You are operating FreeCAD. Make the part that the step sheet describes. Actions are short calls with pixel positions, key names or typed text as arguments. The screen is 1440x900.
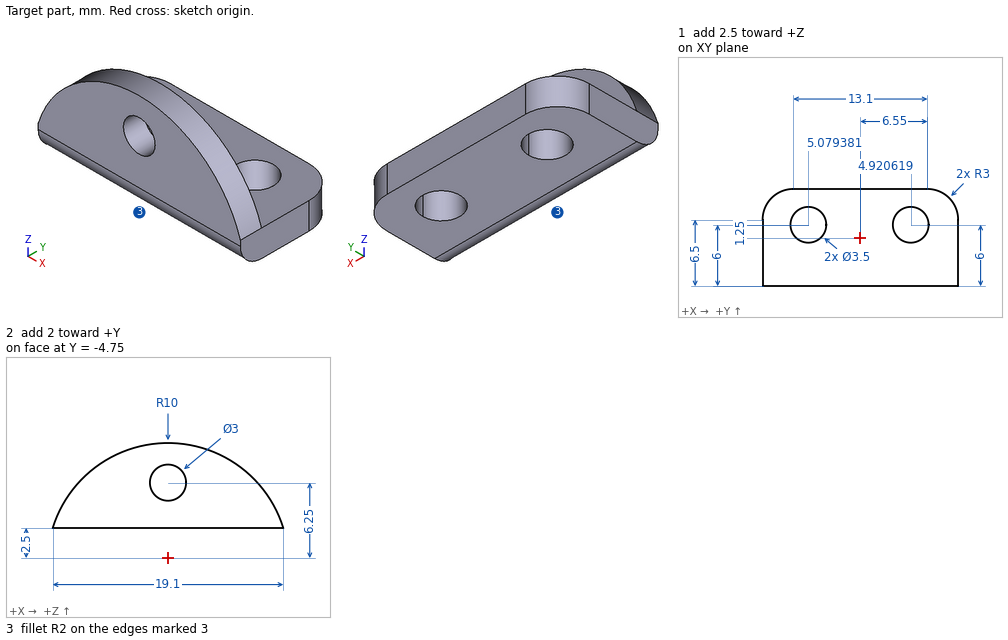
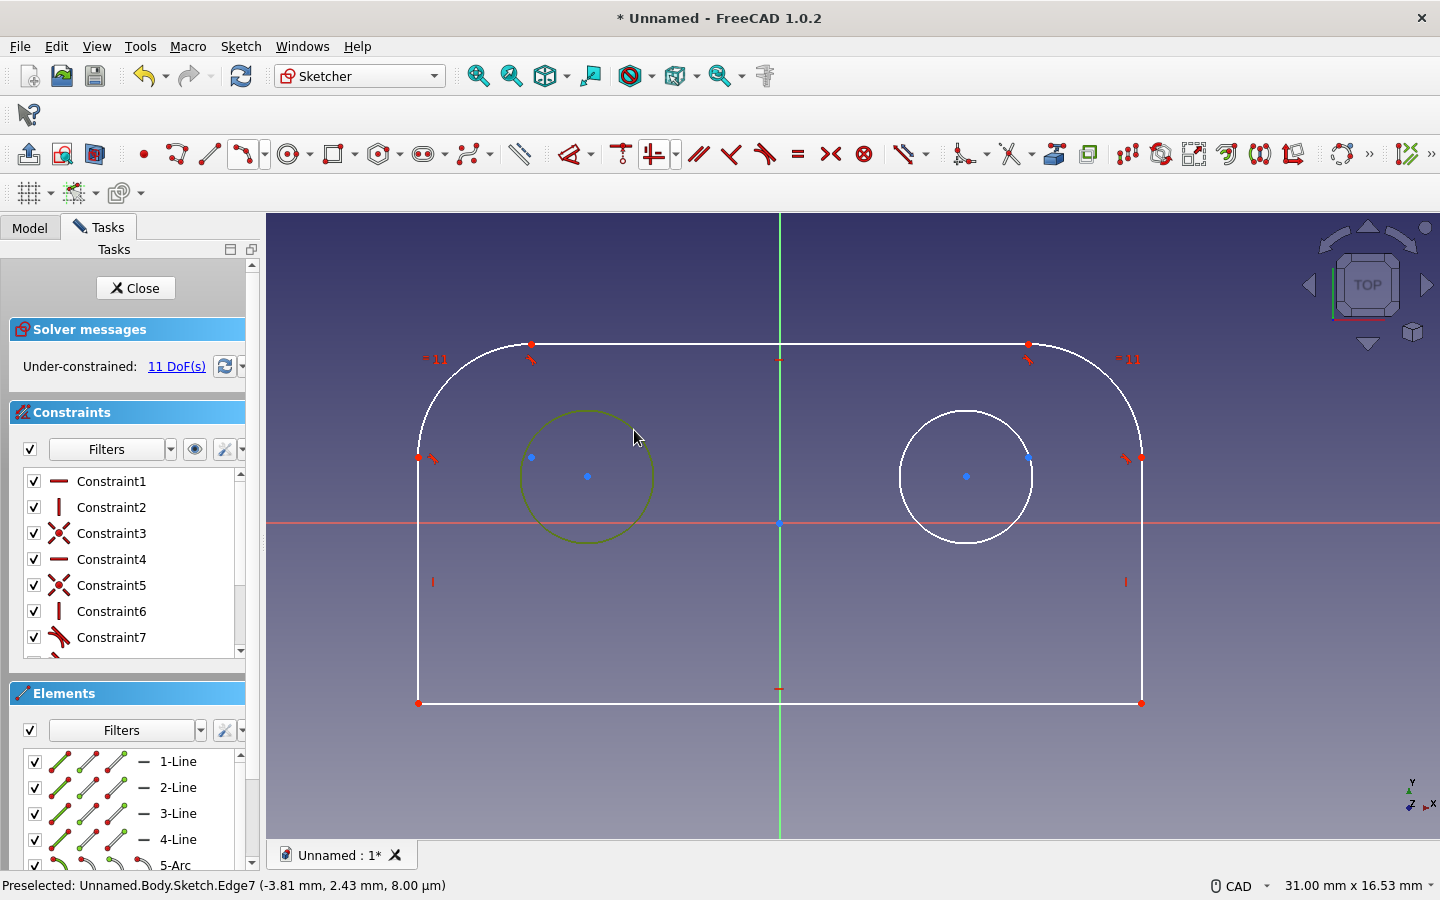
click(1013, 430)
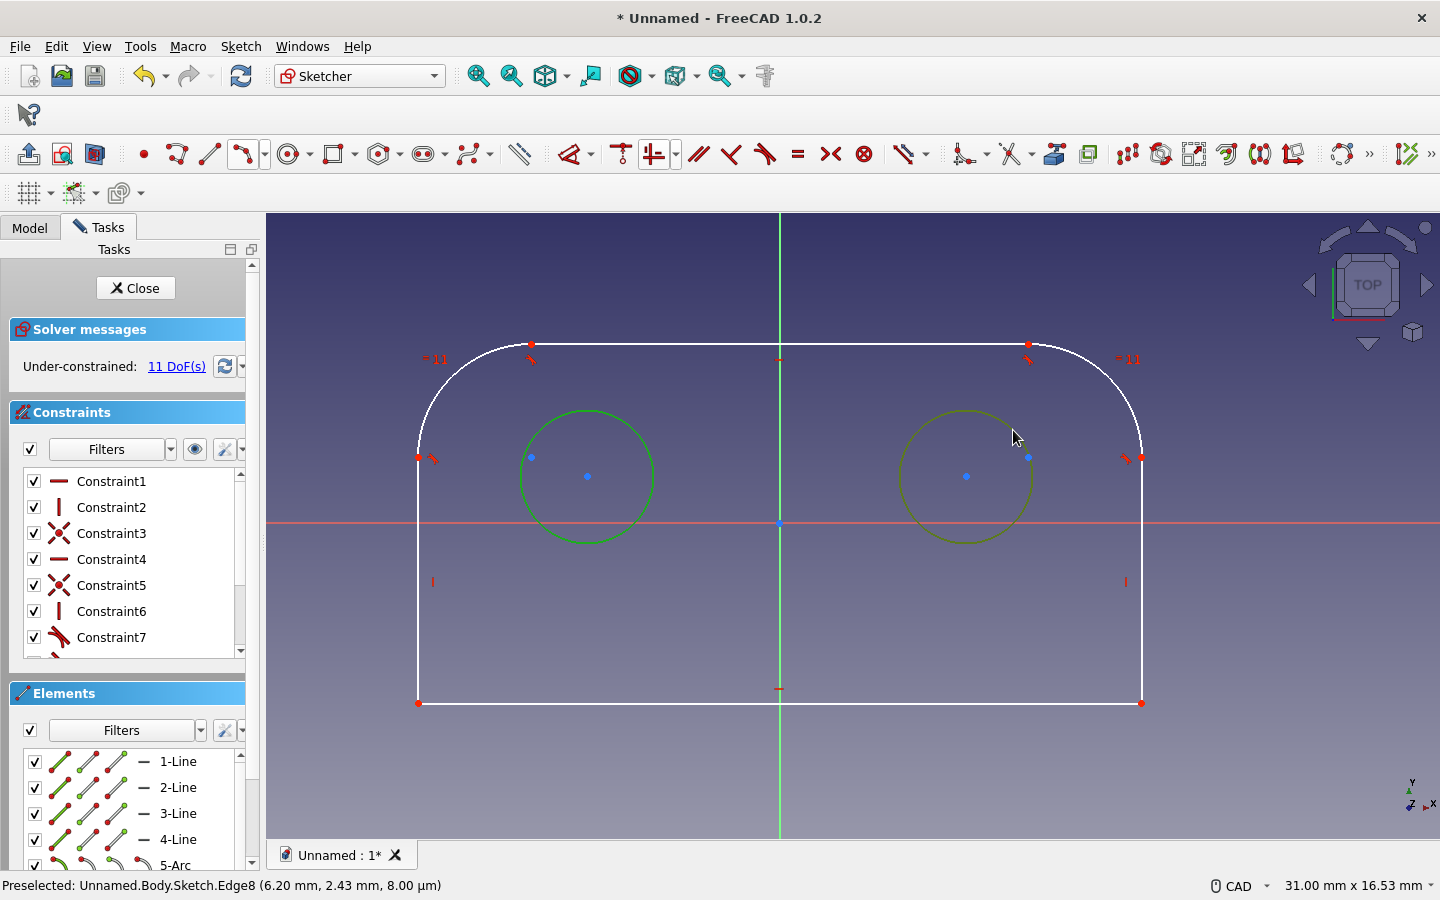
click(798, 154)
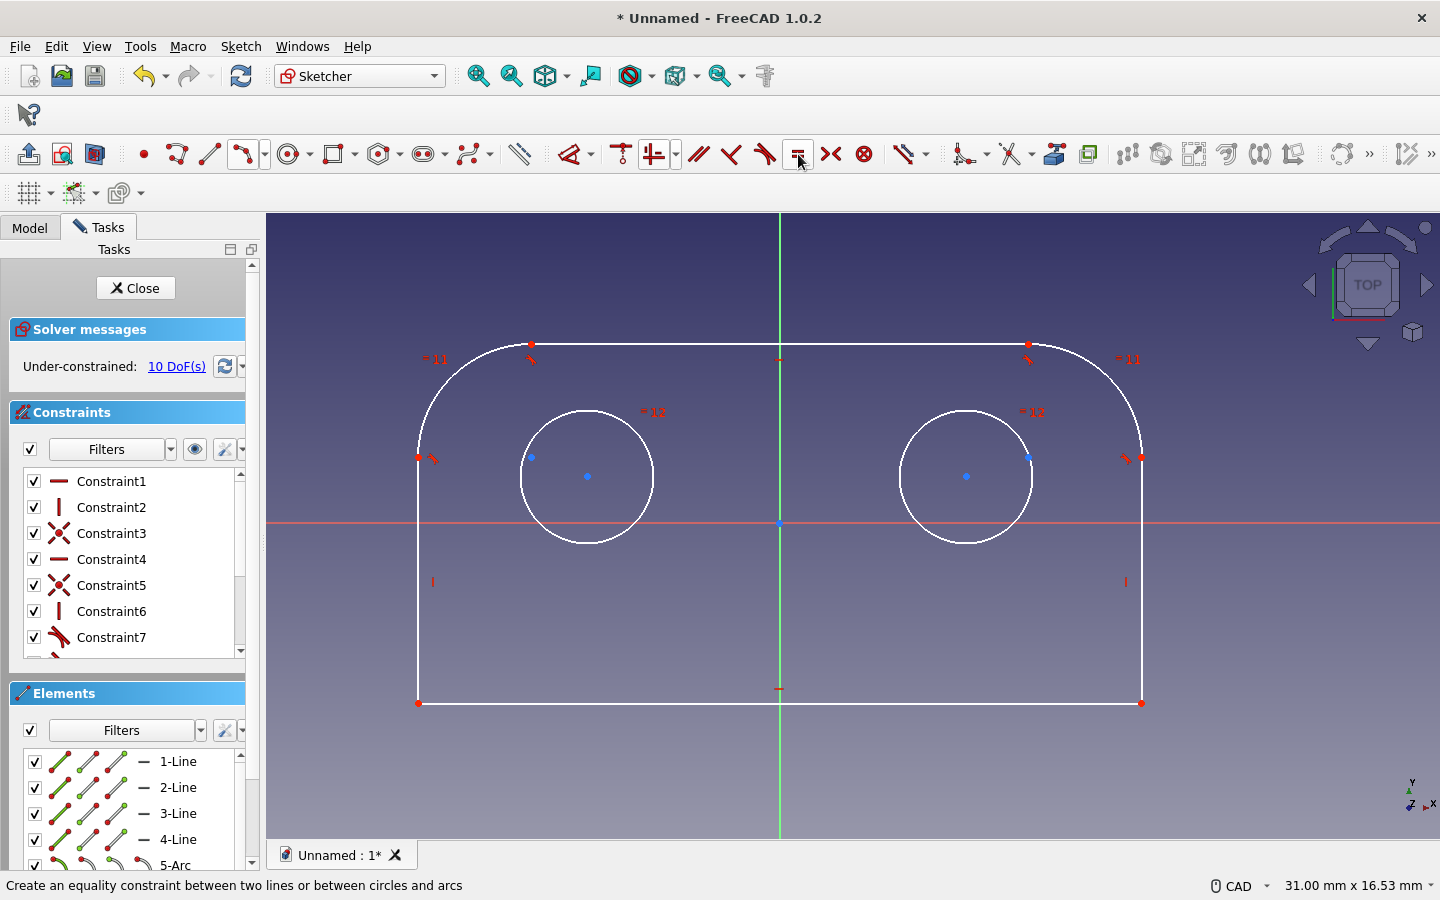
click(568, 154)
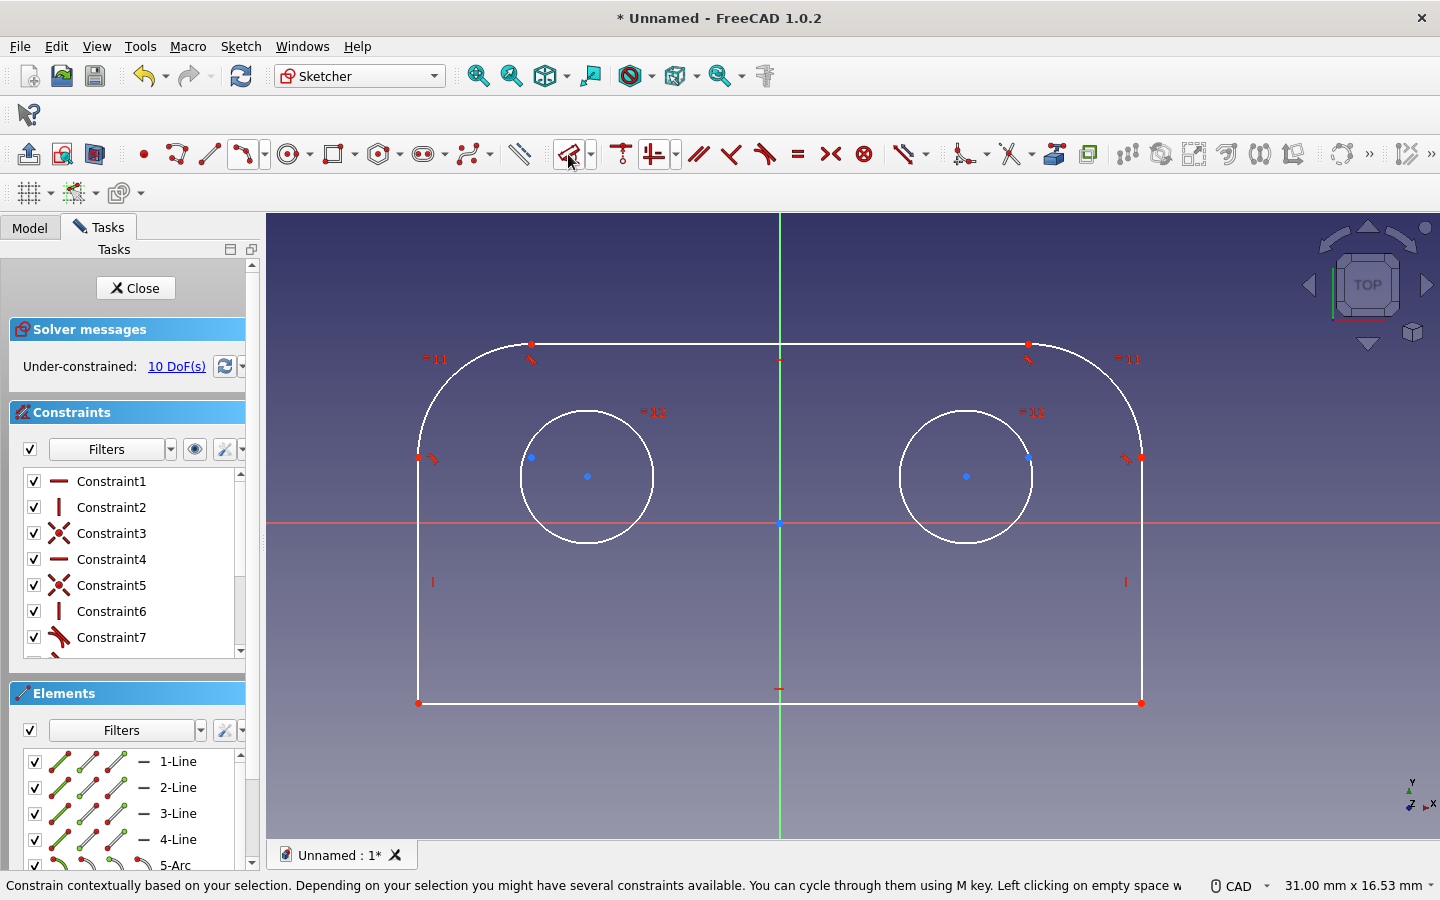
click(480, 356)
click(465, 327)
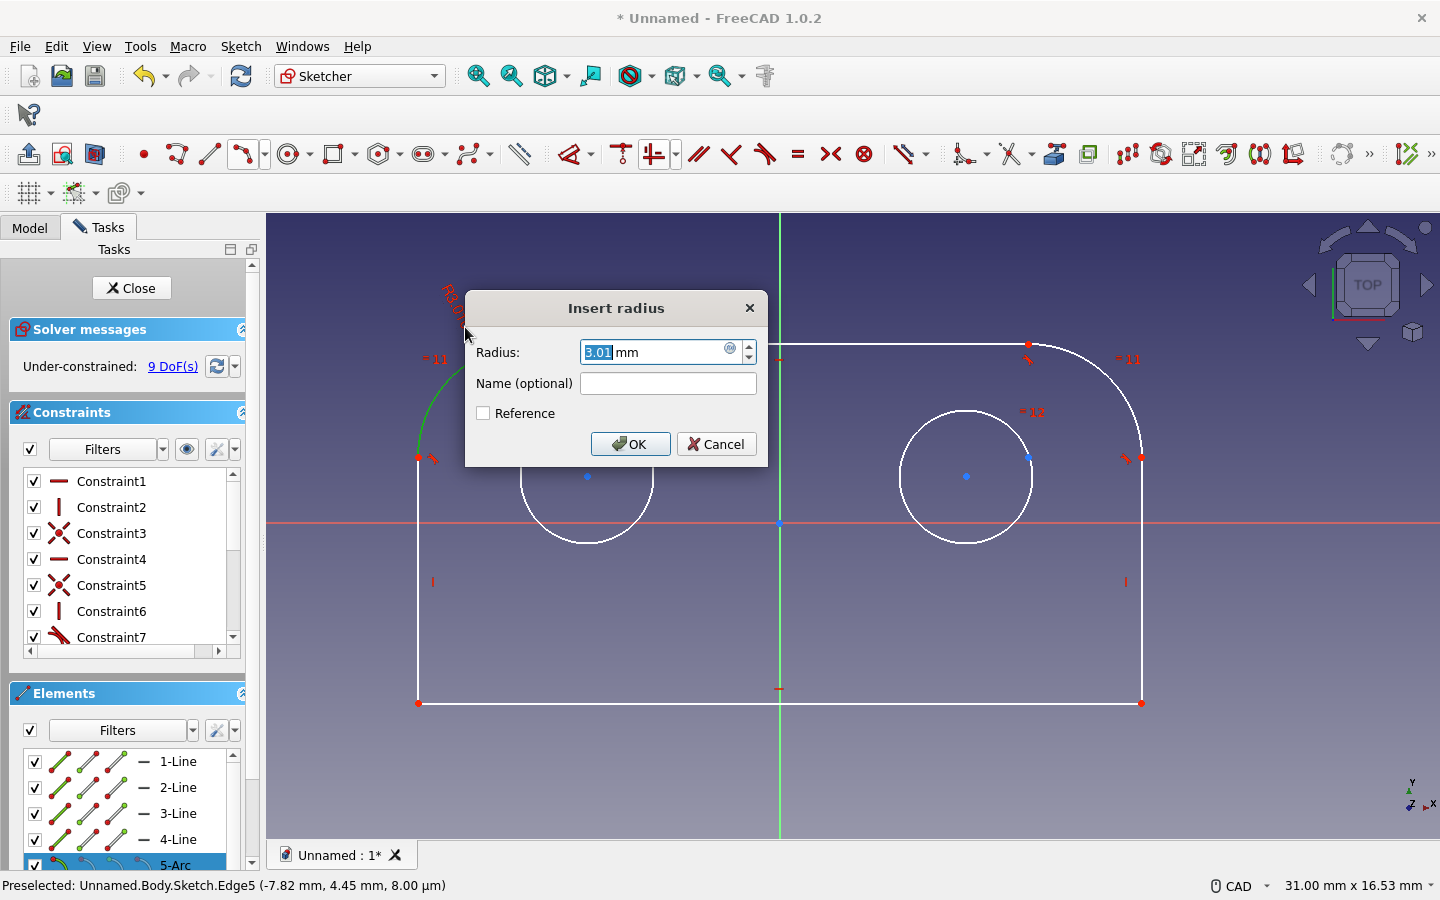
text(3)
key(Return)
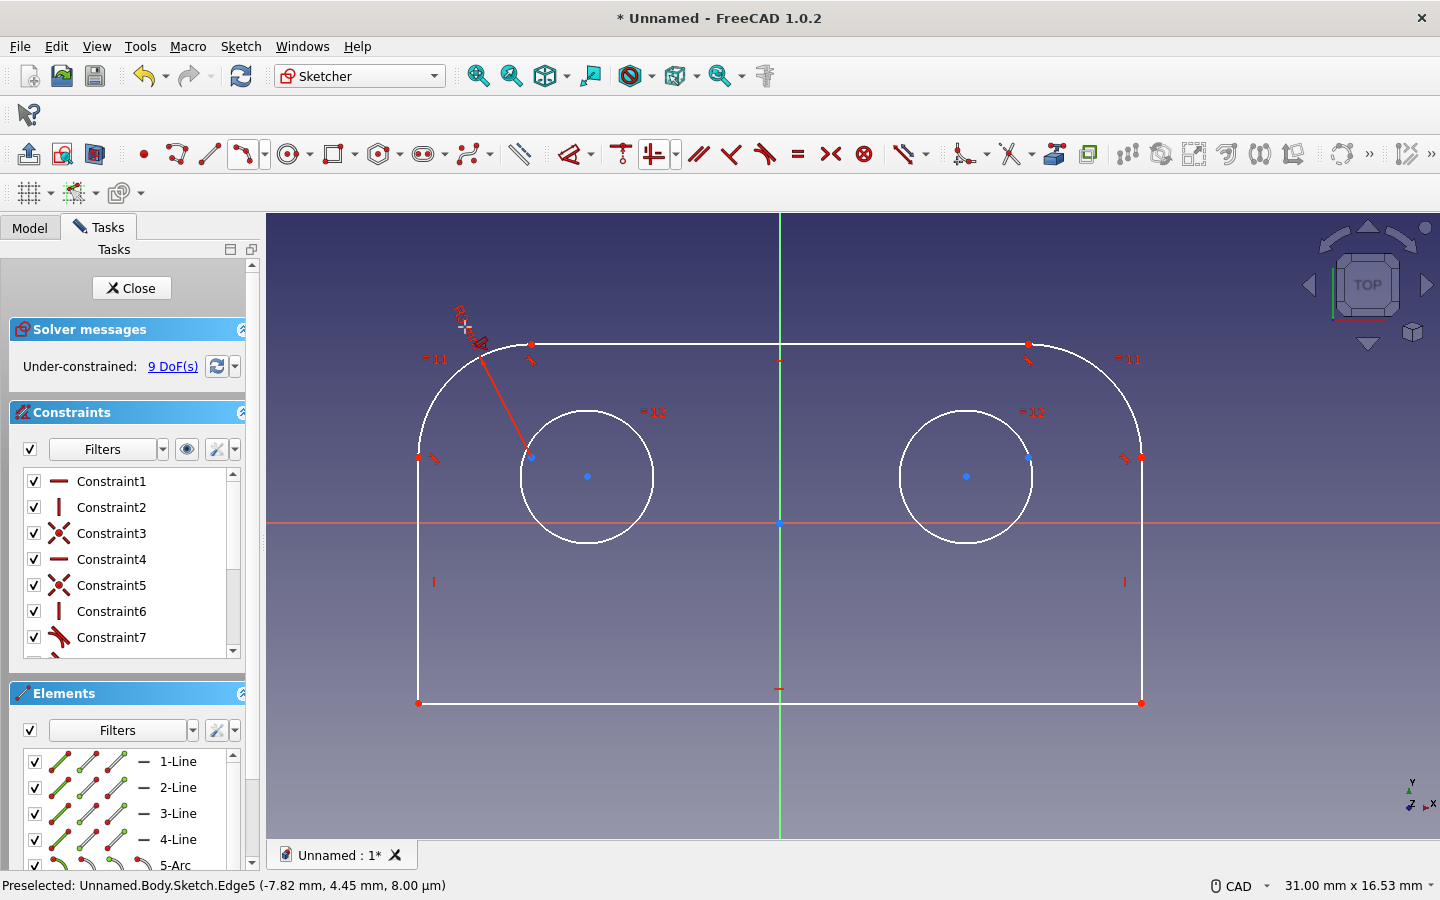
click(634, 430)
click(657, 407)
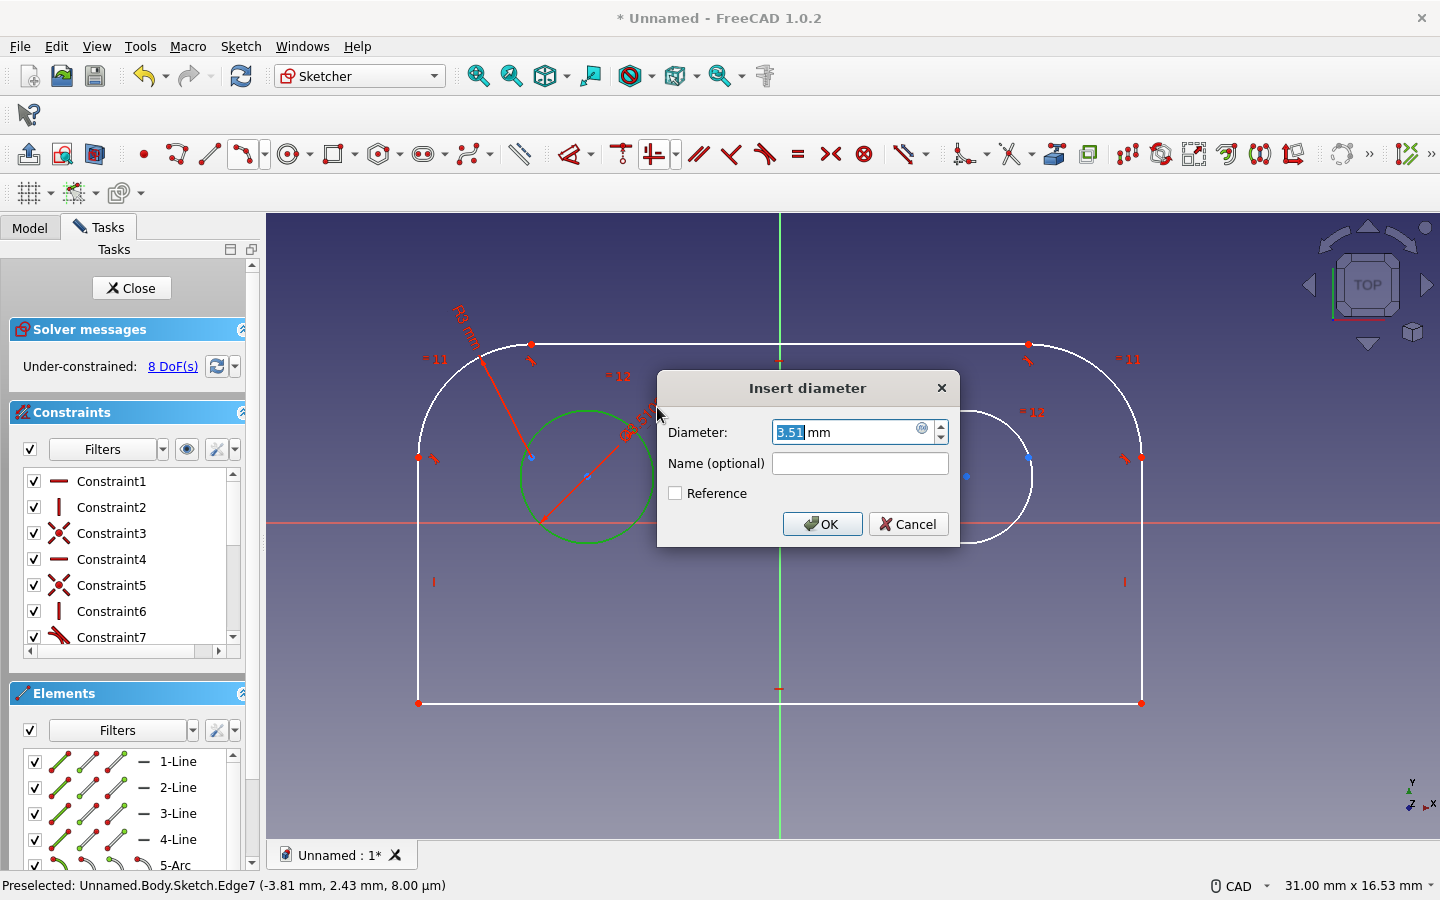
text(3.5)
key(Return)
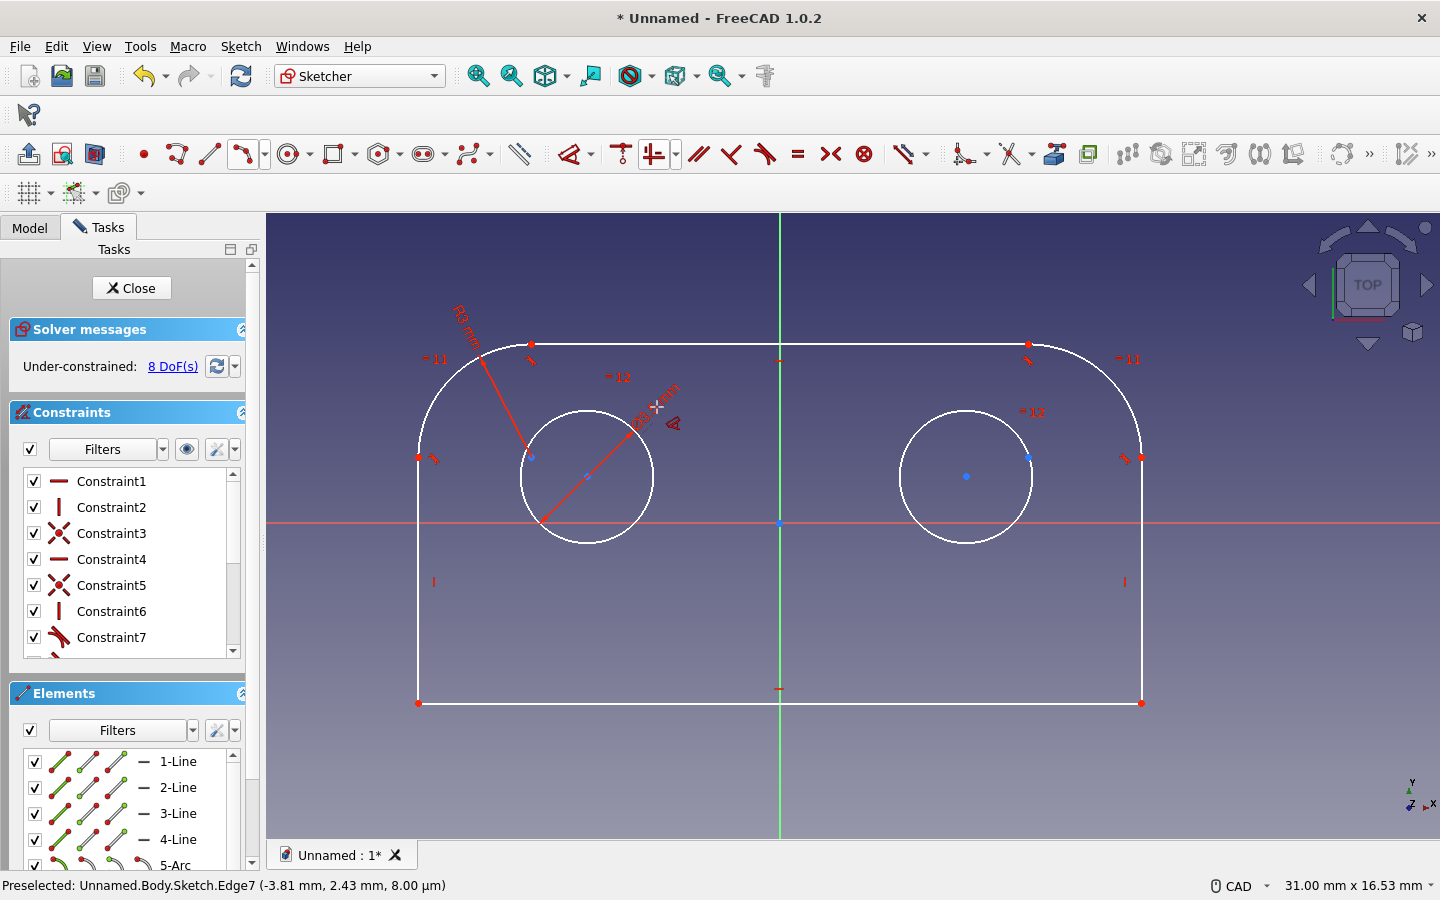
click(418, 704)